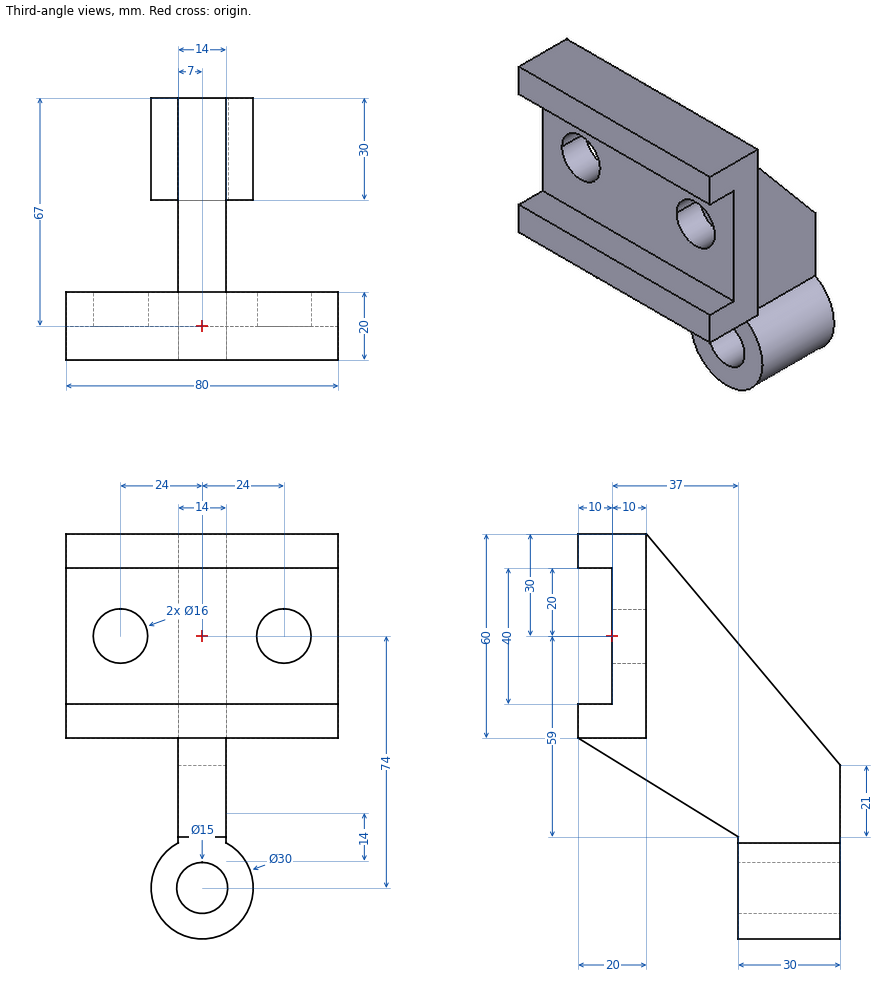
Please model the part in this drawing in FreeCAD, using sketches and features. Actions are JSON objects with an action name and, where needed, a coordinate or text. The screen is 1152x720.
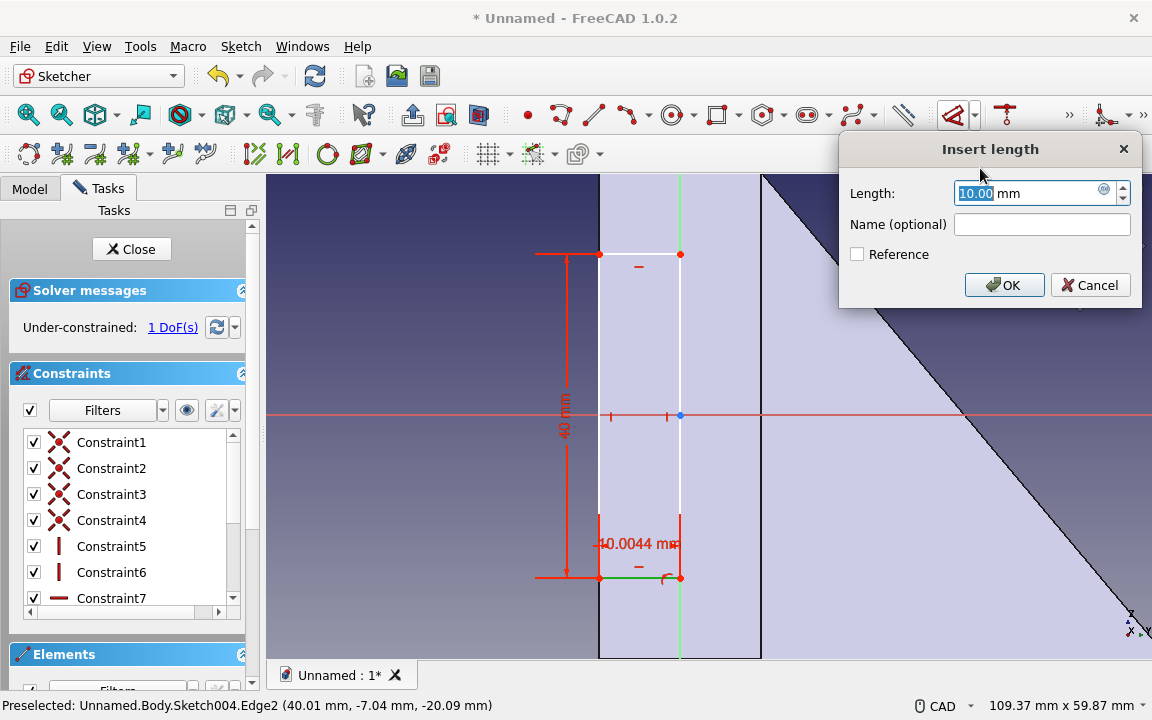
{"action": "type", "text": "10"}
{"action": "key", "text": "Return"}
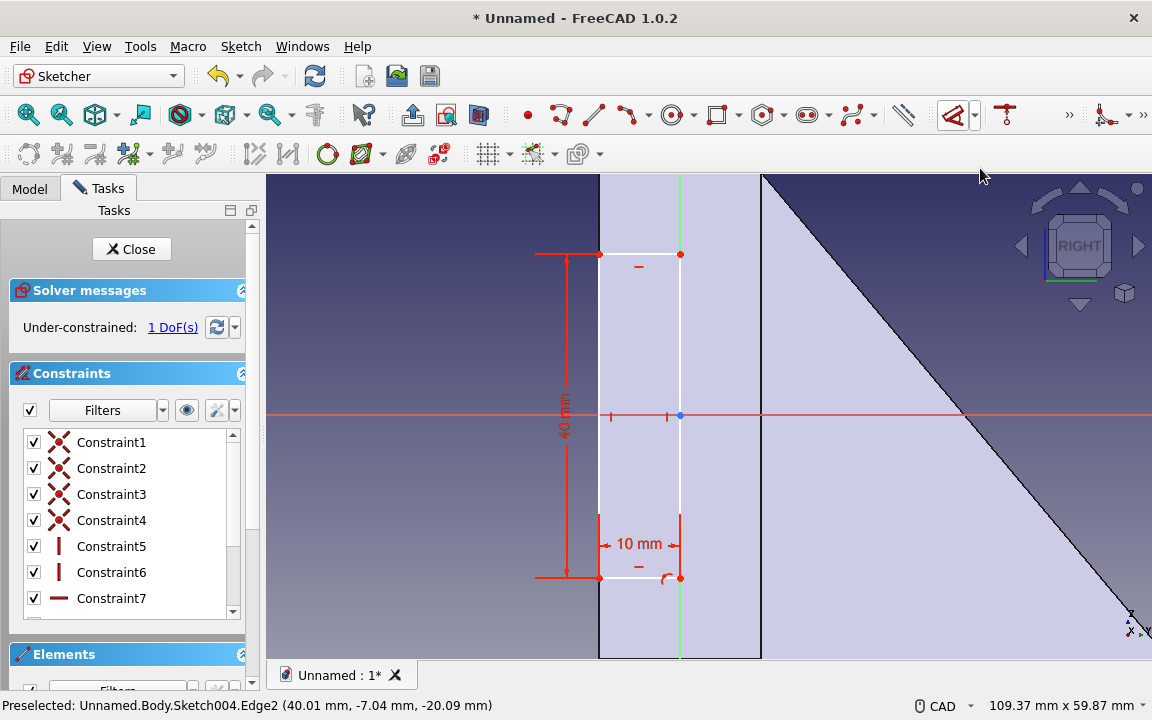
{"action": "left_click", "coordinate": [599, 254]}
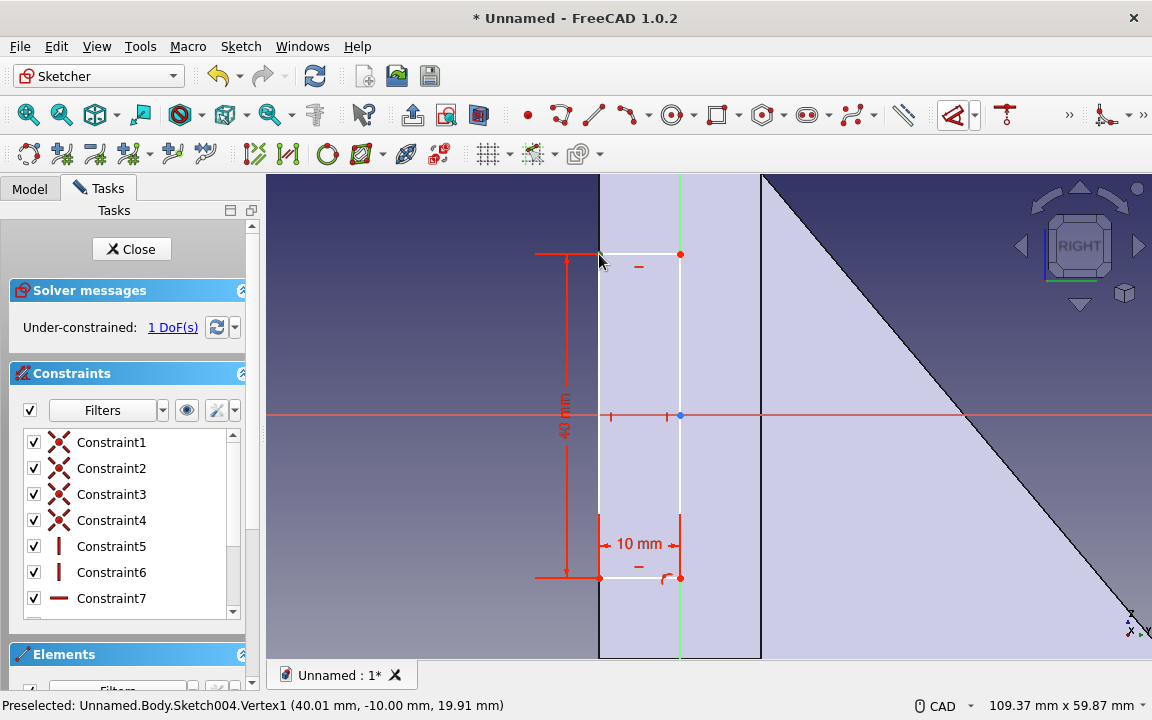
{"action": "left_click", "coordinate": [974, 116]}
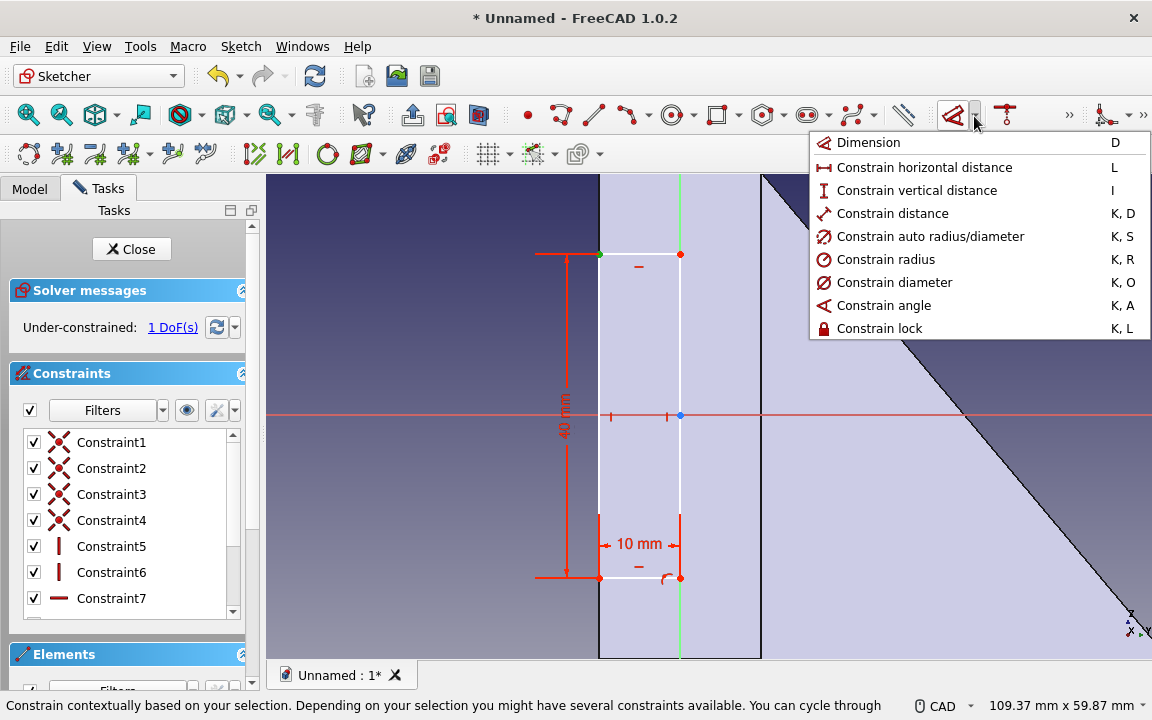
{"action": "left_click", "coordinate": [980, 190]}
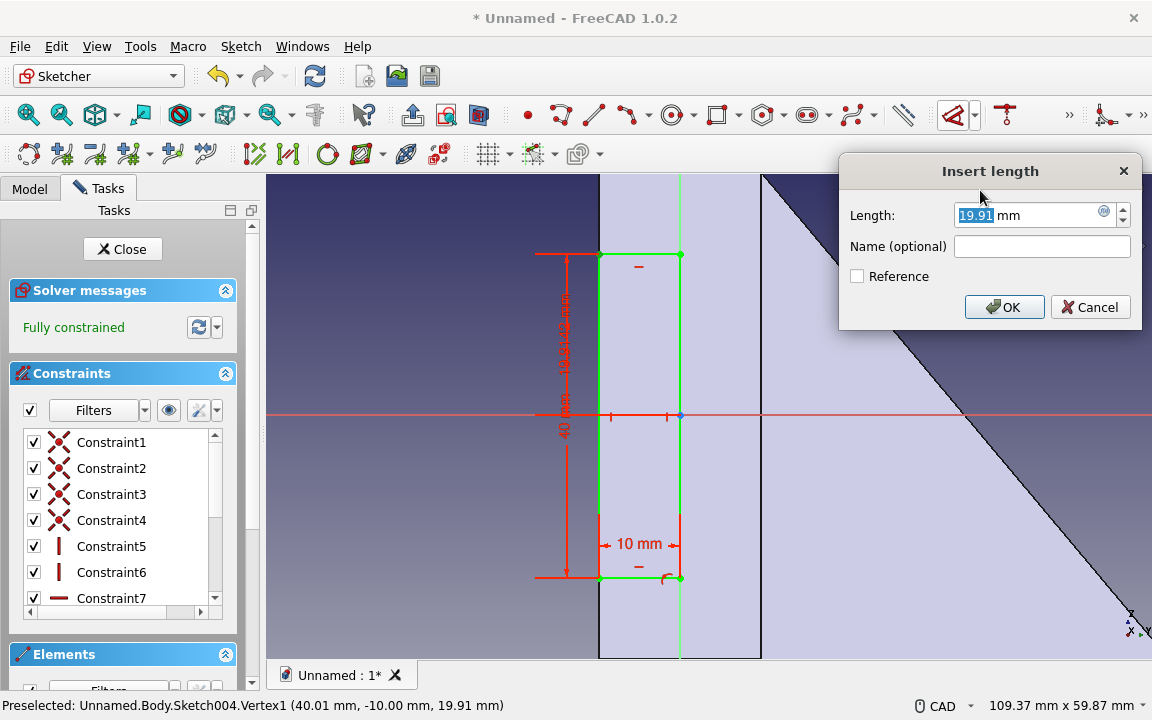
{"action": "type", "text": "20"}
{"action": "key", "text": "Return"}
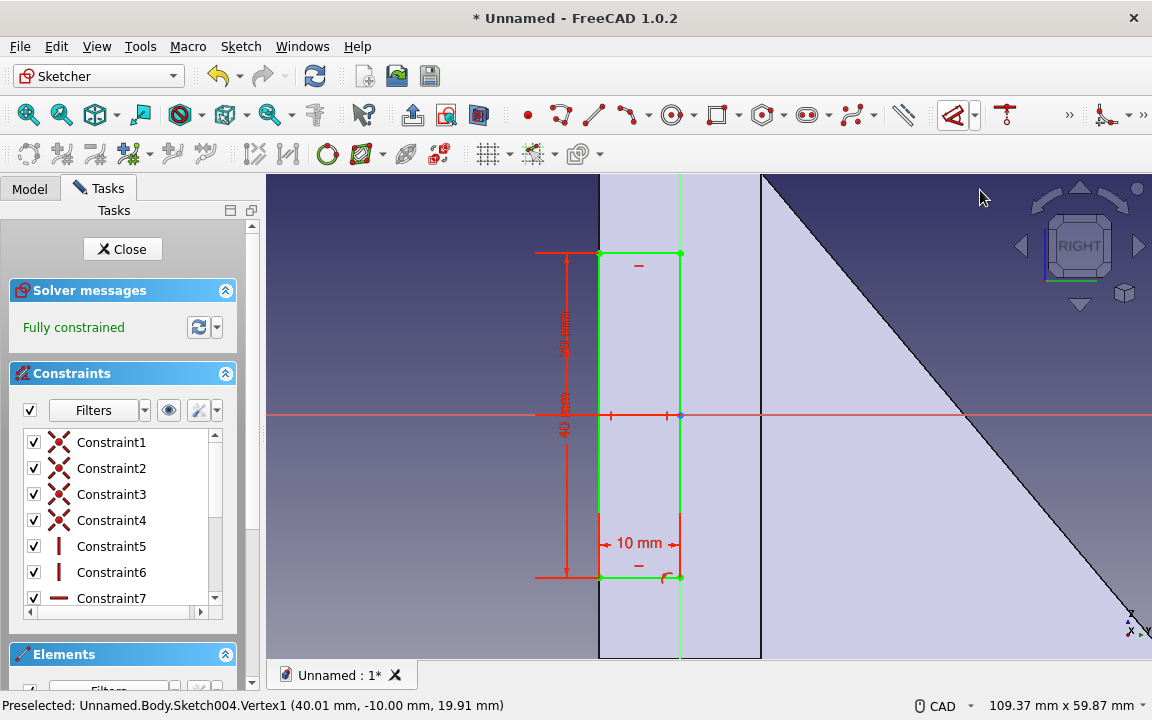
{"action": "left_click", "coordinate": [123, 249]}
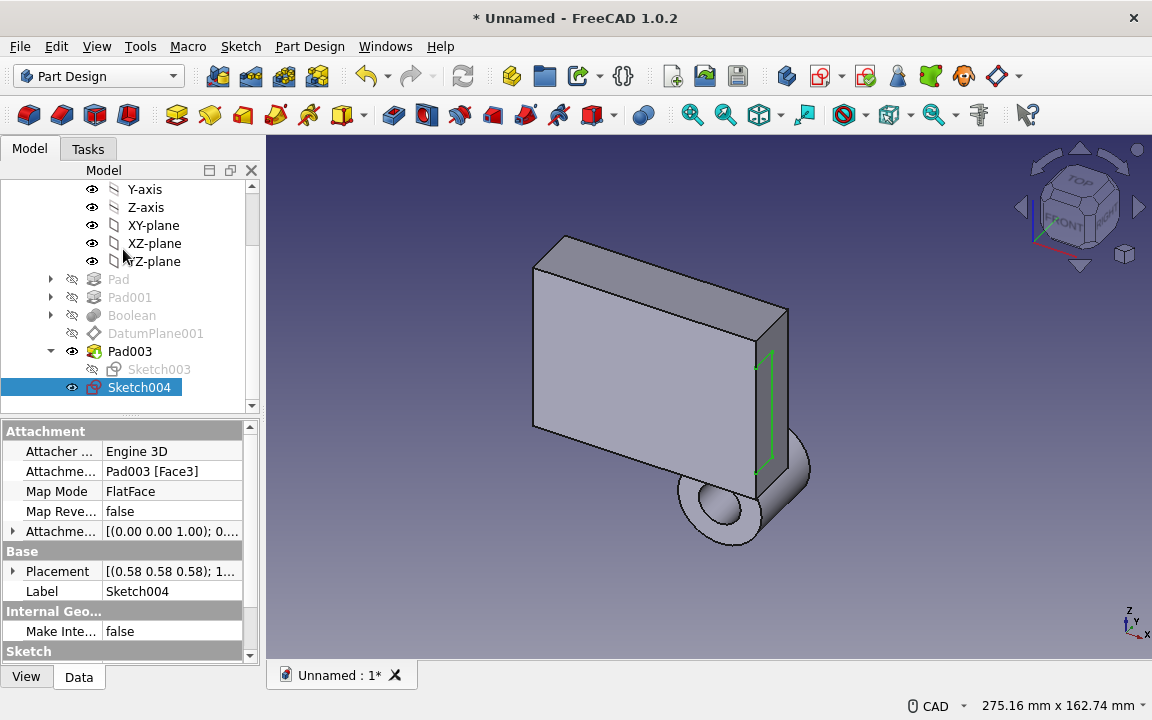
{"action": "left_click", "coordinate": [394, 116]}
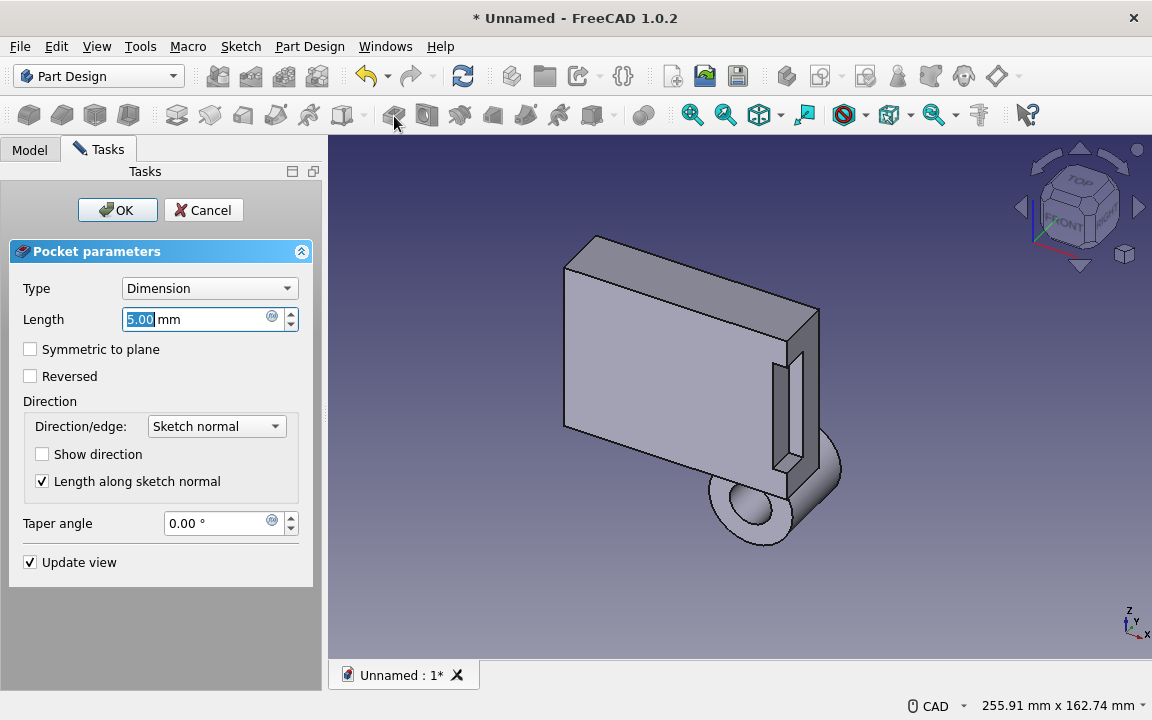
{"action": "left_click", "coordinate": [210, 288]}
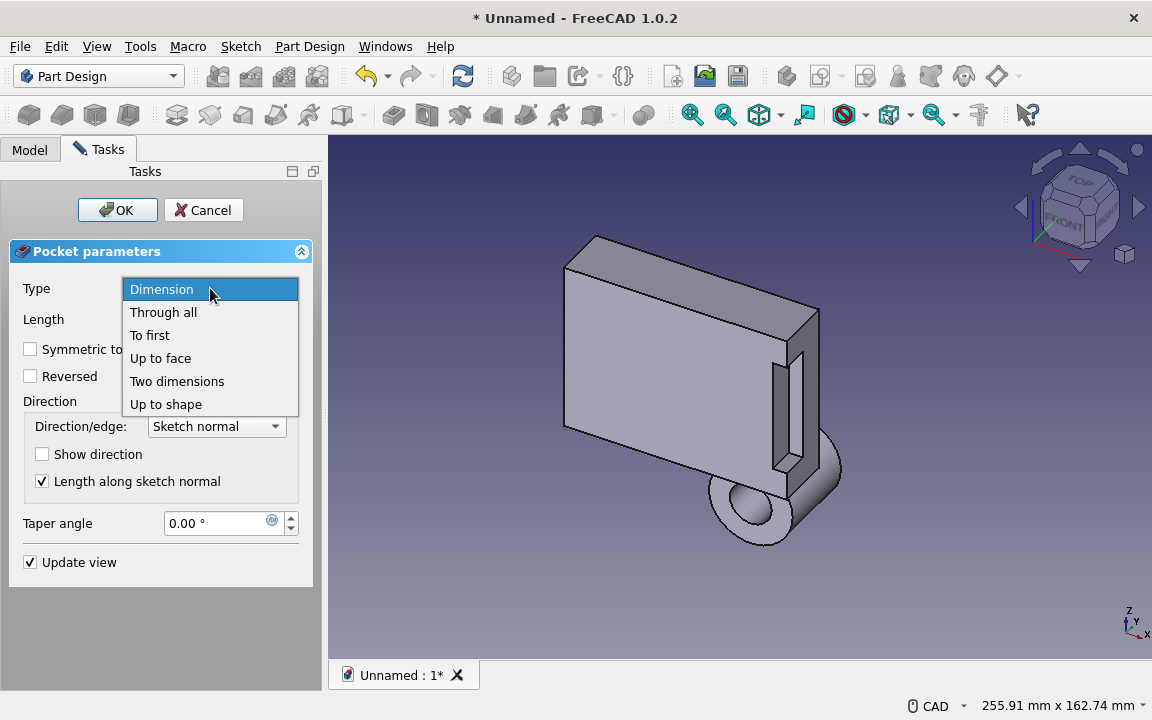
{"action": "left_click", "coordinate": [208, 312]}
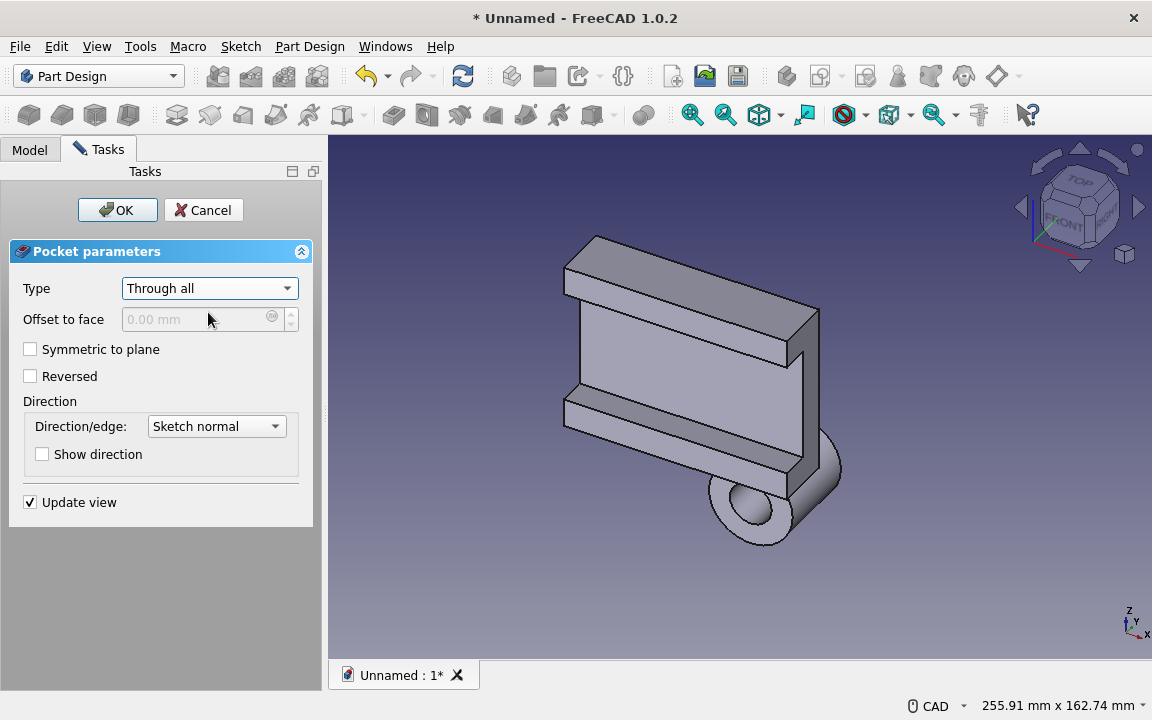
{"action": "left_click", "coordinate": [118, 210]}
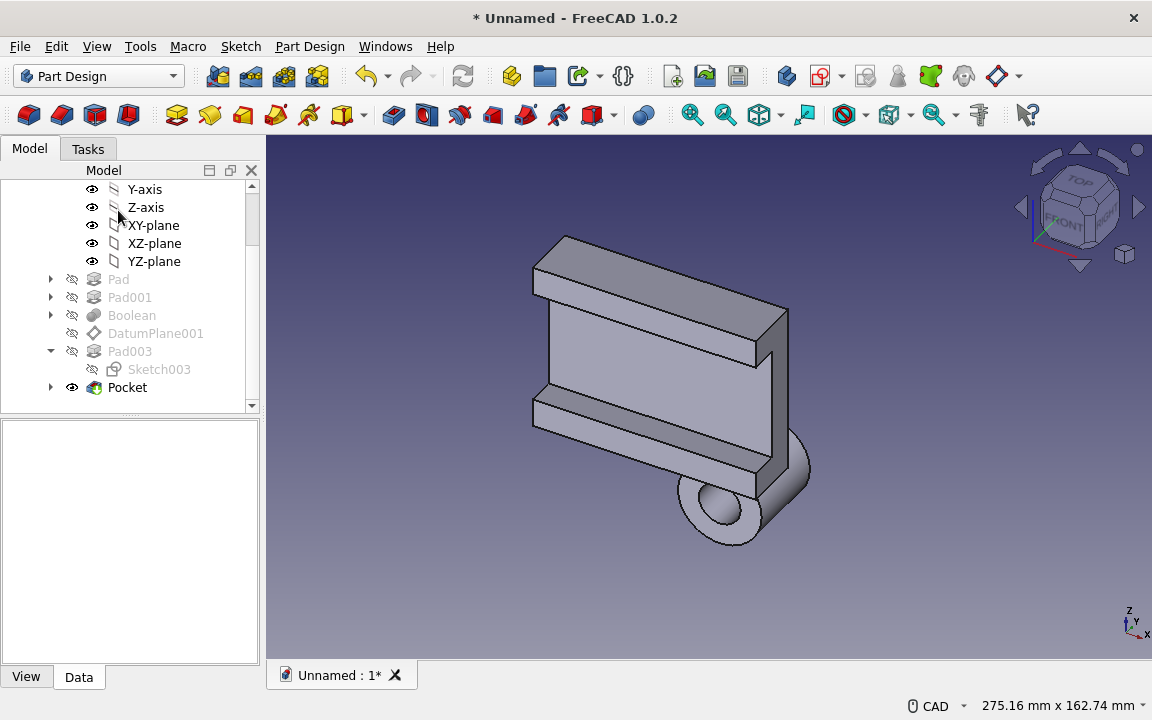
{"action": "key", "text": "4"}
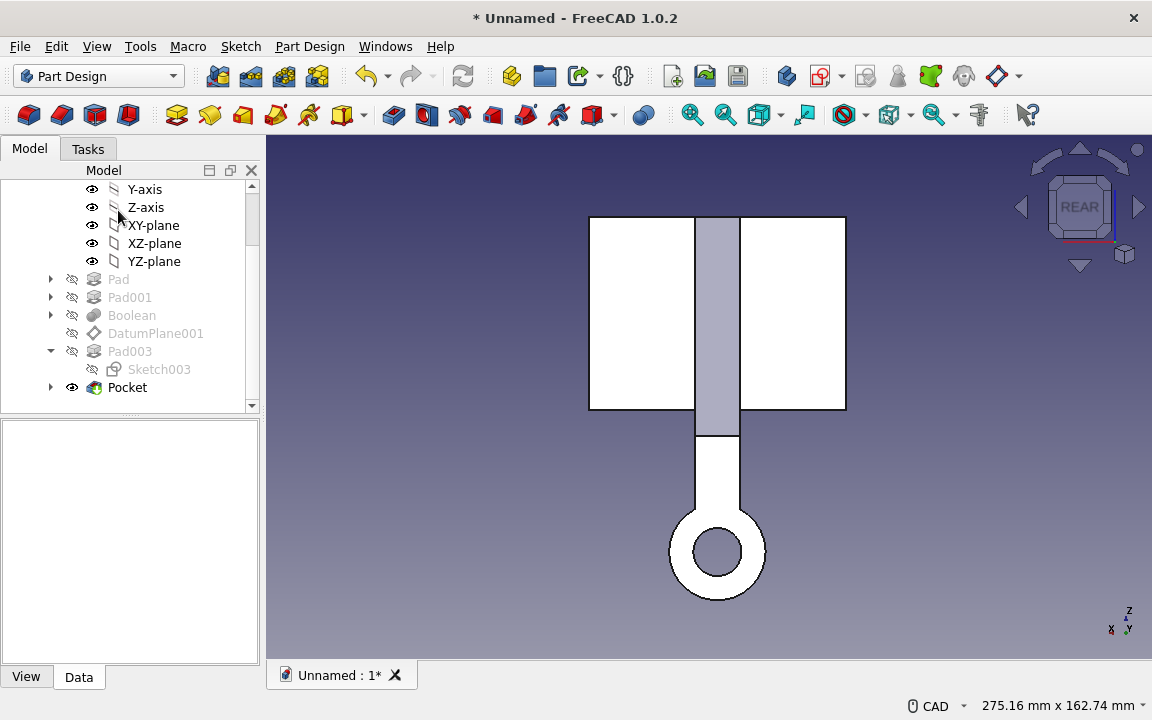
{"action": "left_click", "coordinate": [793, 285]}